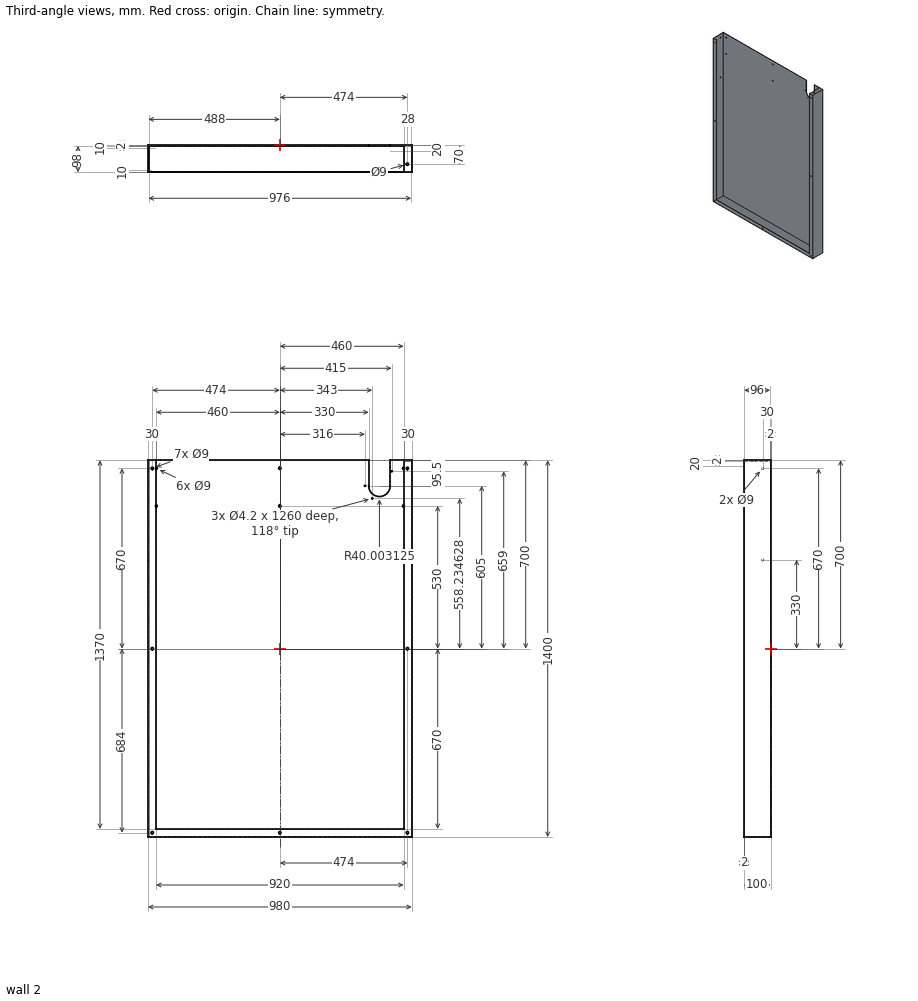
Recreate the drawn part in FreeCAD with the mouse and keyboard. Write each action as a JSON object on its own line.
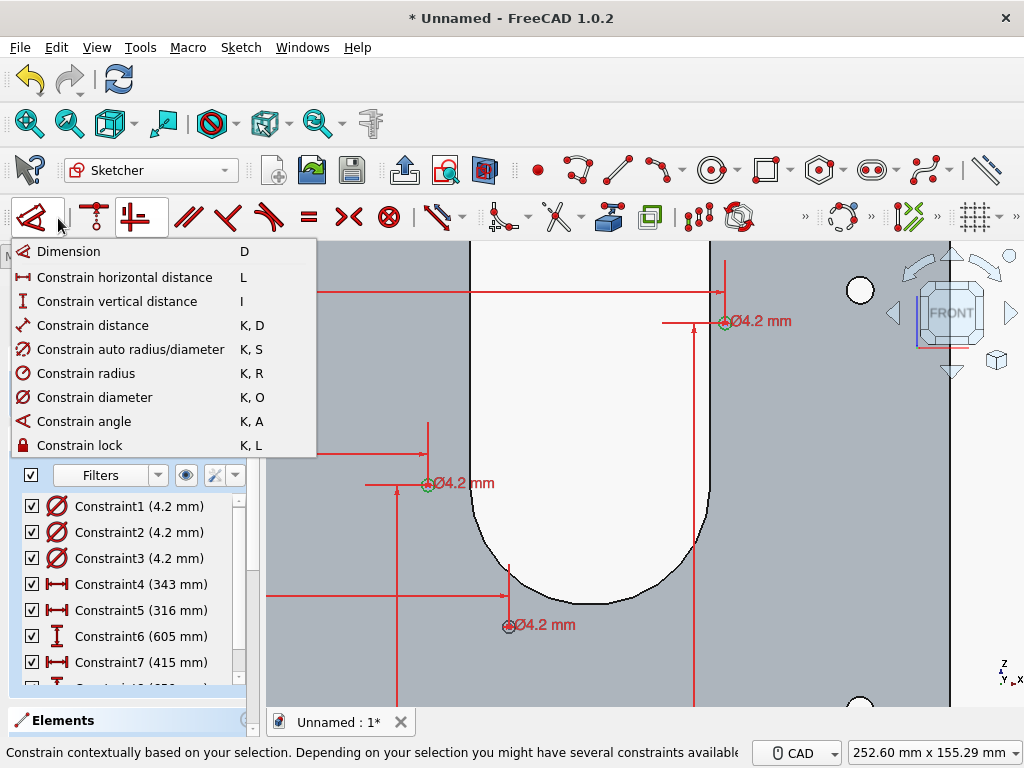
{"action": "left_click", "coordinate": [164, 301]}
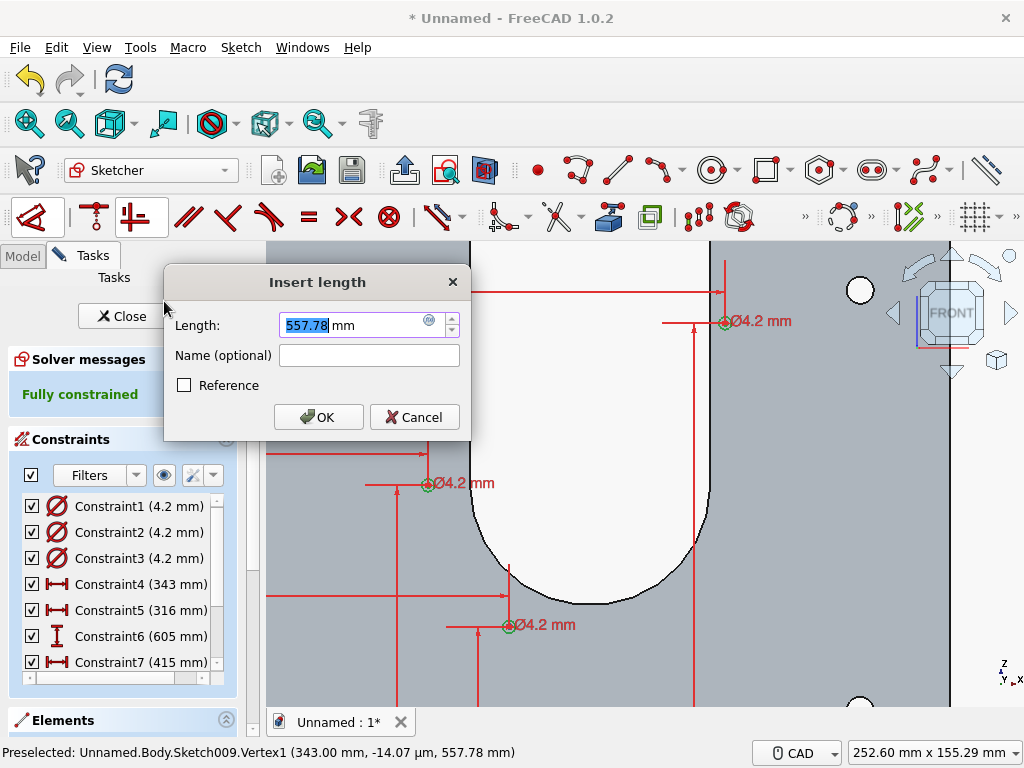
{"action": "type", "text": "558.234628"}
{"action": "key", "text": "Return"}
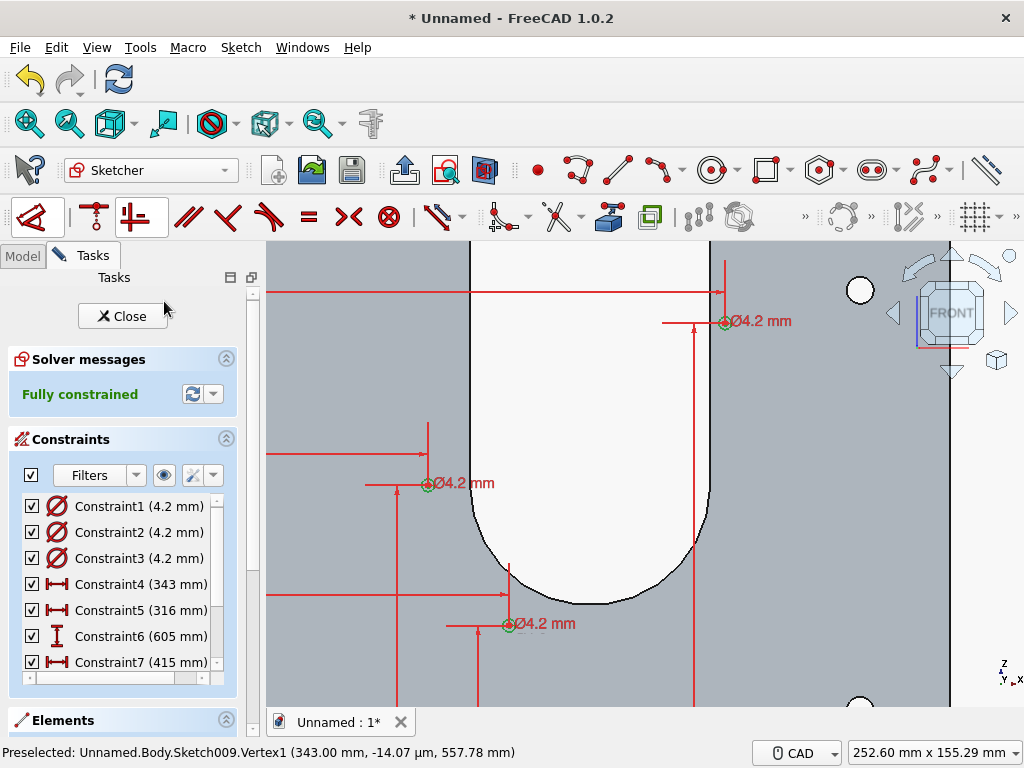
{"action": "left_click", "coordinate": [123, 316]}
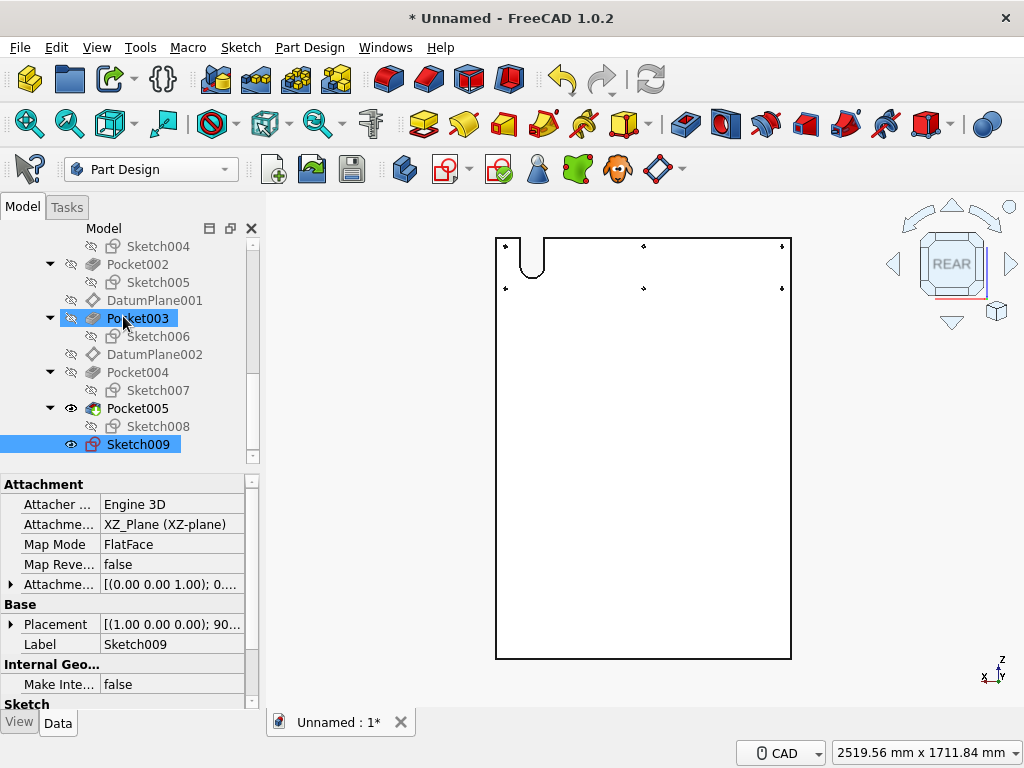
{"action": "left_click", "coordinate": [726, 124]}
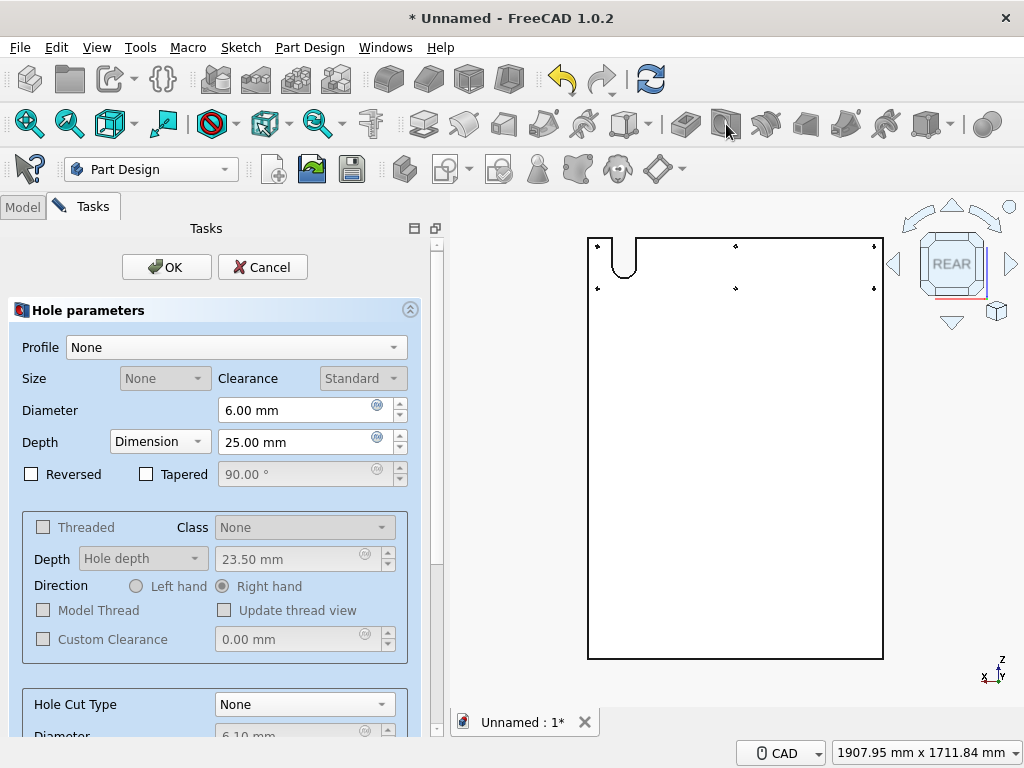
{"action": "triple_click", "coordinate": [305, 410]}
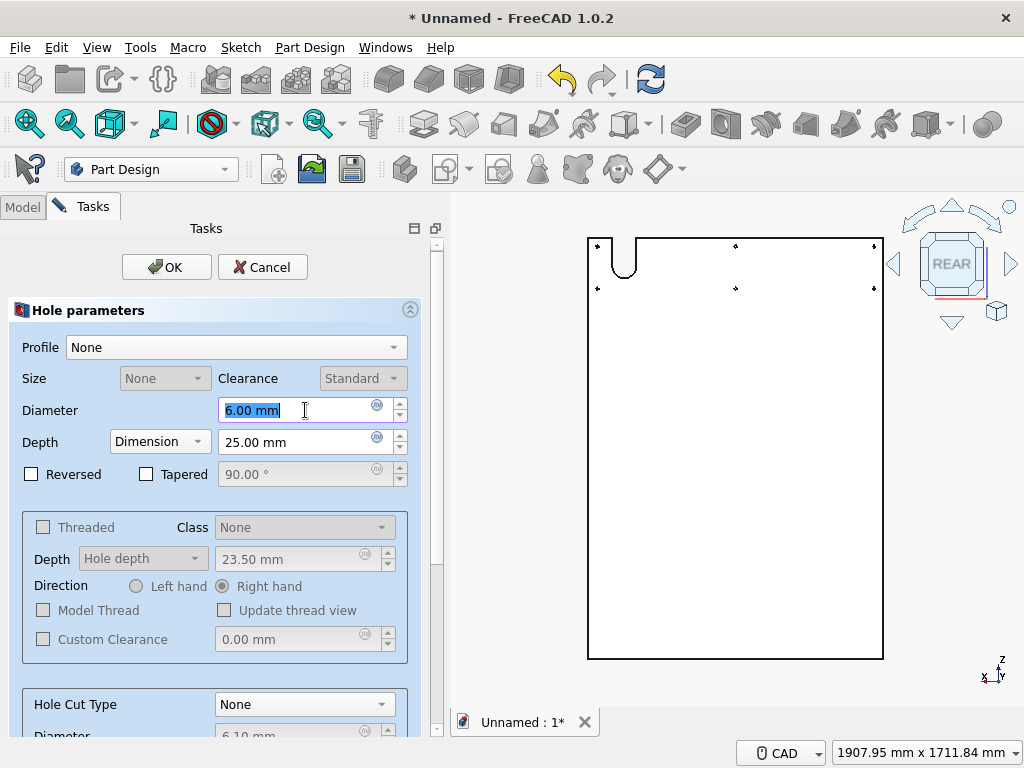
{"action": "type", "text": "4.2"}
{"action": "key", "text": "Tab"}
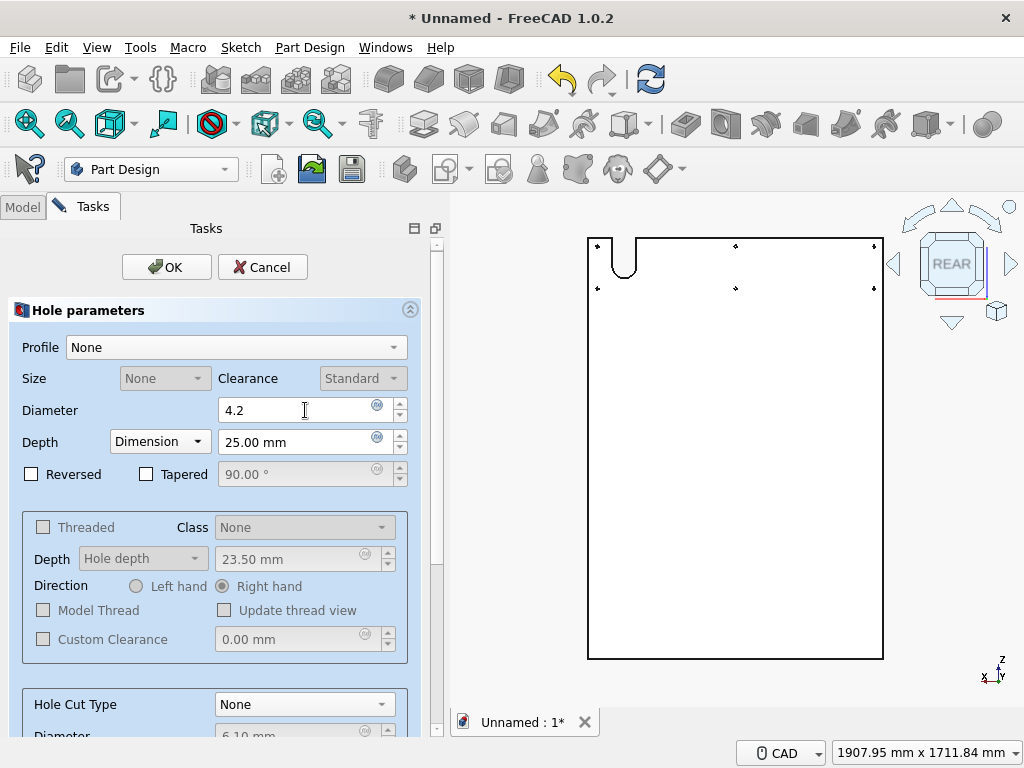
{"action": "triple_click", "coordinate": [305, 442]}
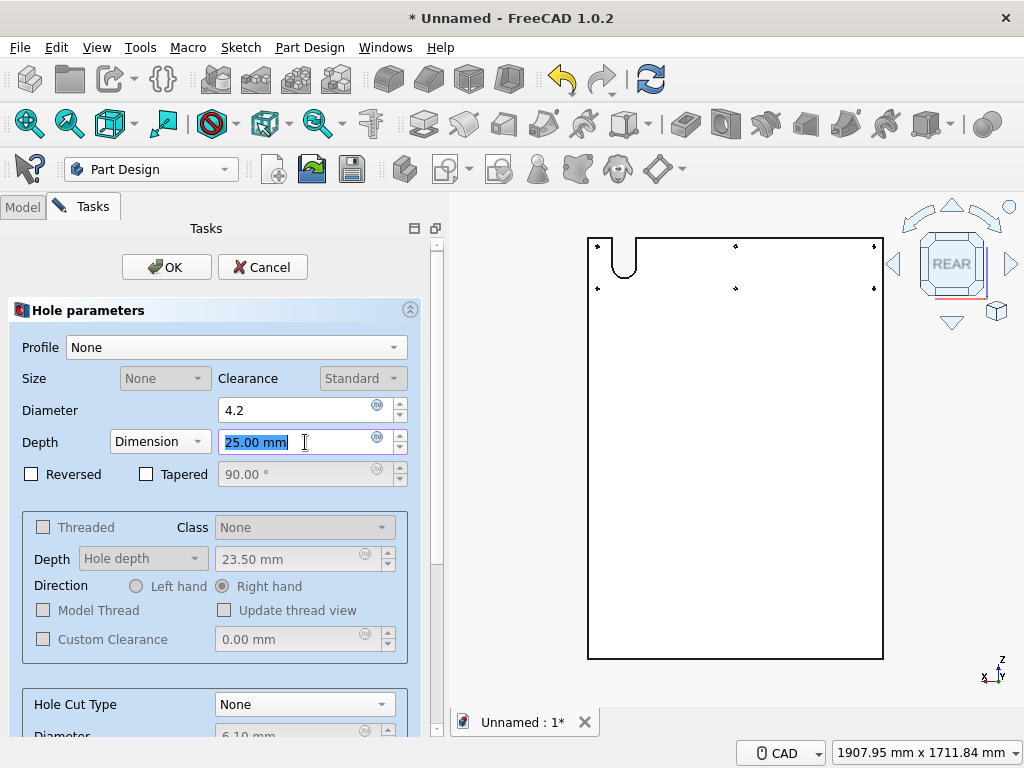
{"action": "type", "text": "1260"}
{"action": "key", "text": "Tab"}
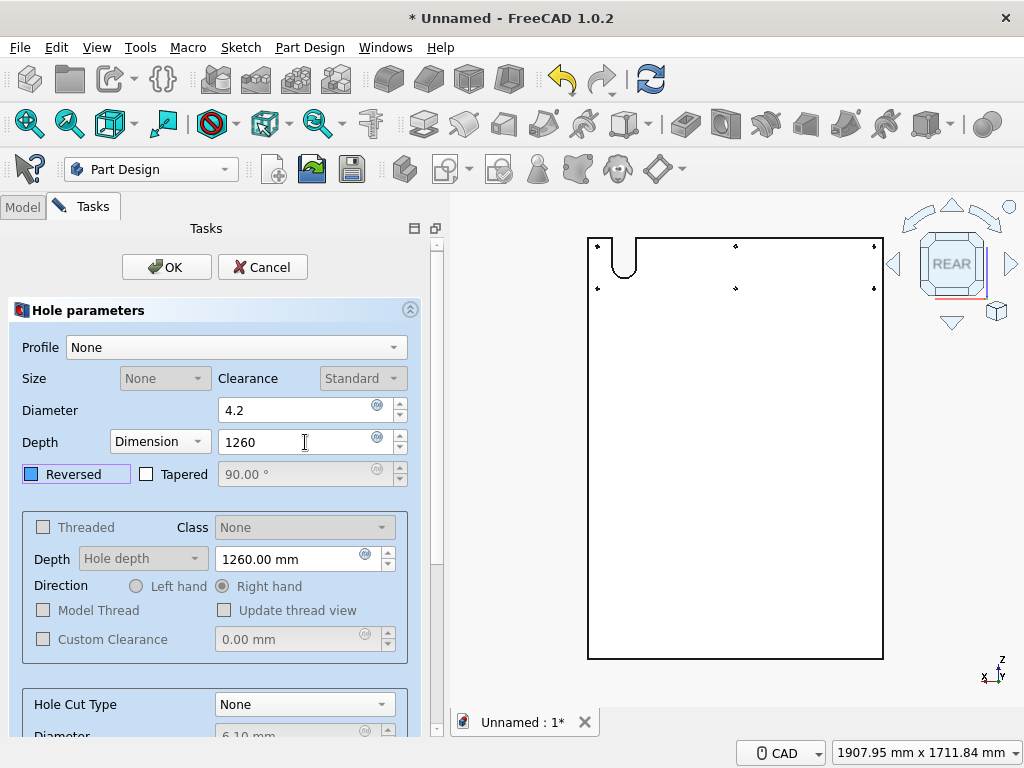
{"action": "left_click", "coordinate": [30, 474]}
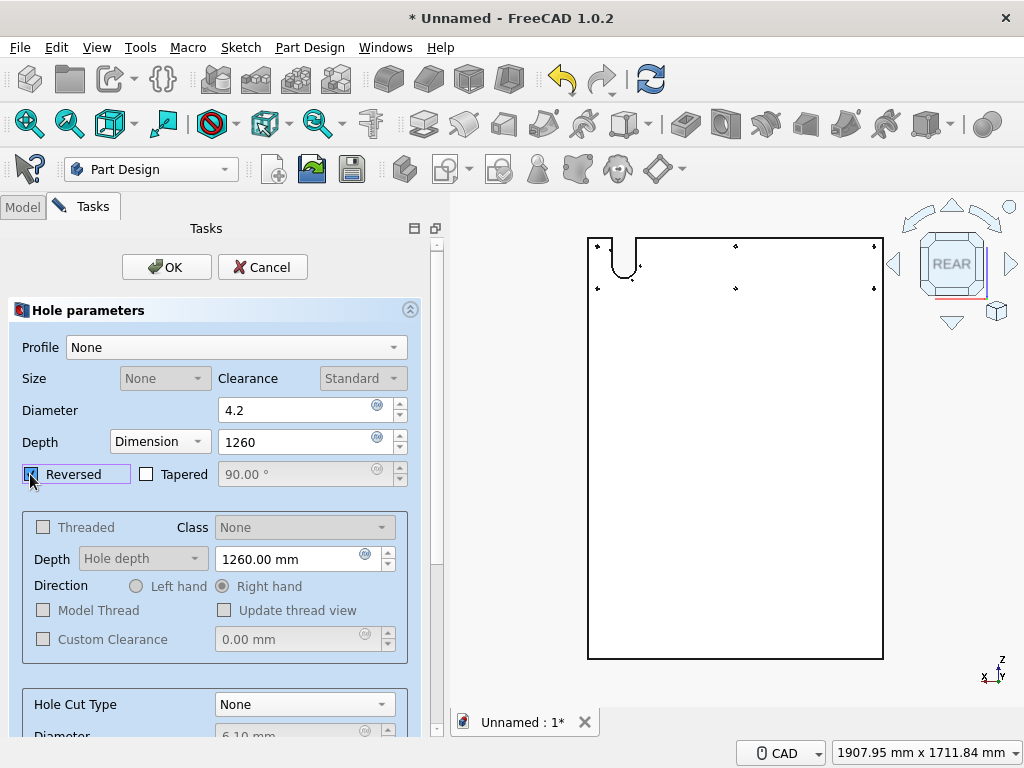
{"action": "left_click", "coordinate": [167, 267]}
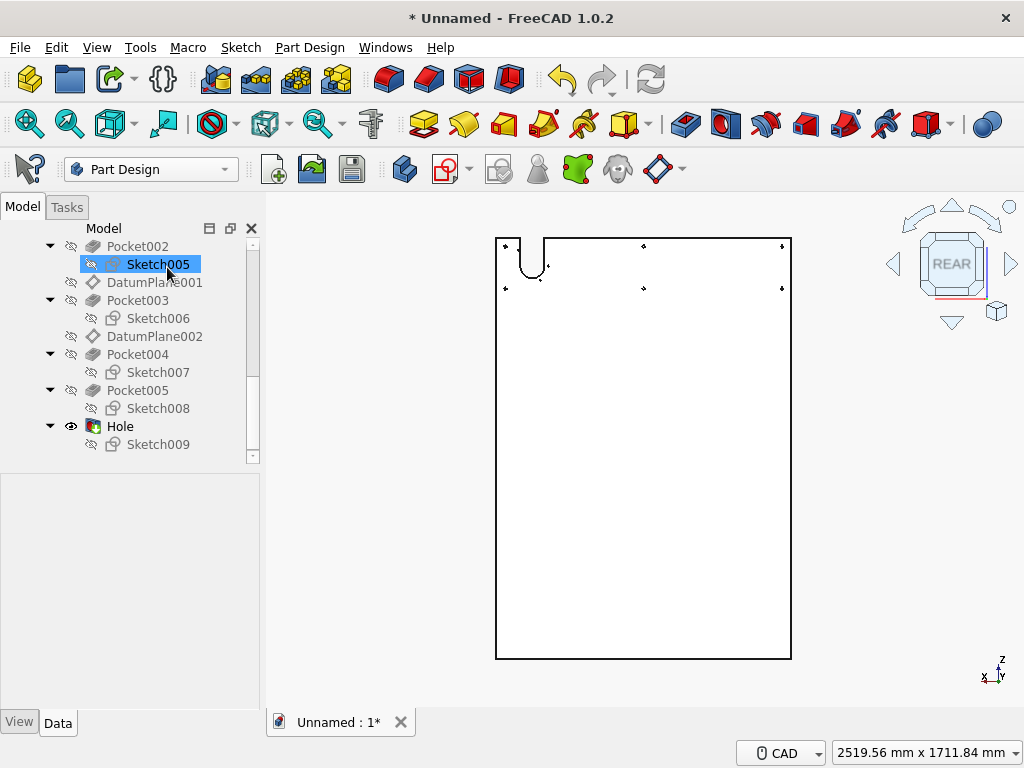
{"action": "key", "text": "0"}